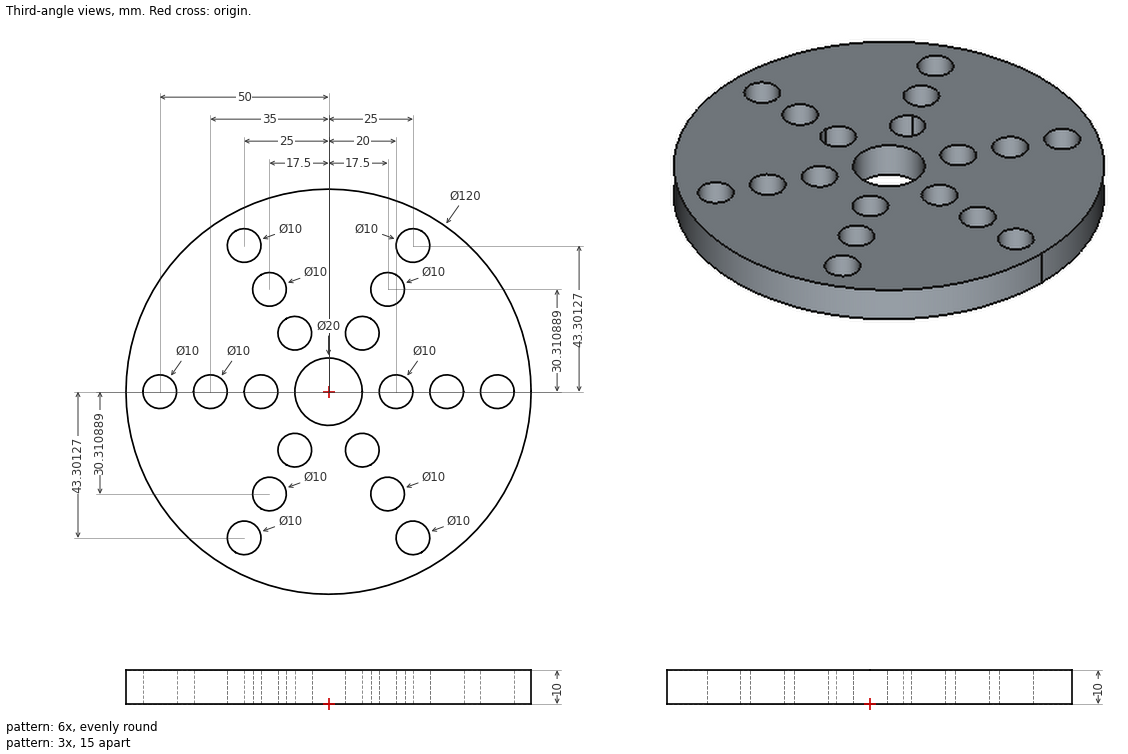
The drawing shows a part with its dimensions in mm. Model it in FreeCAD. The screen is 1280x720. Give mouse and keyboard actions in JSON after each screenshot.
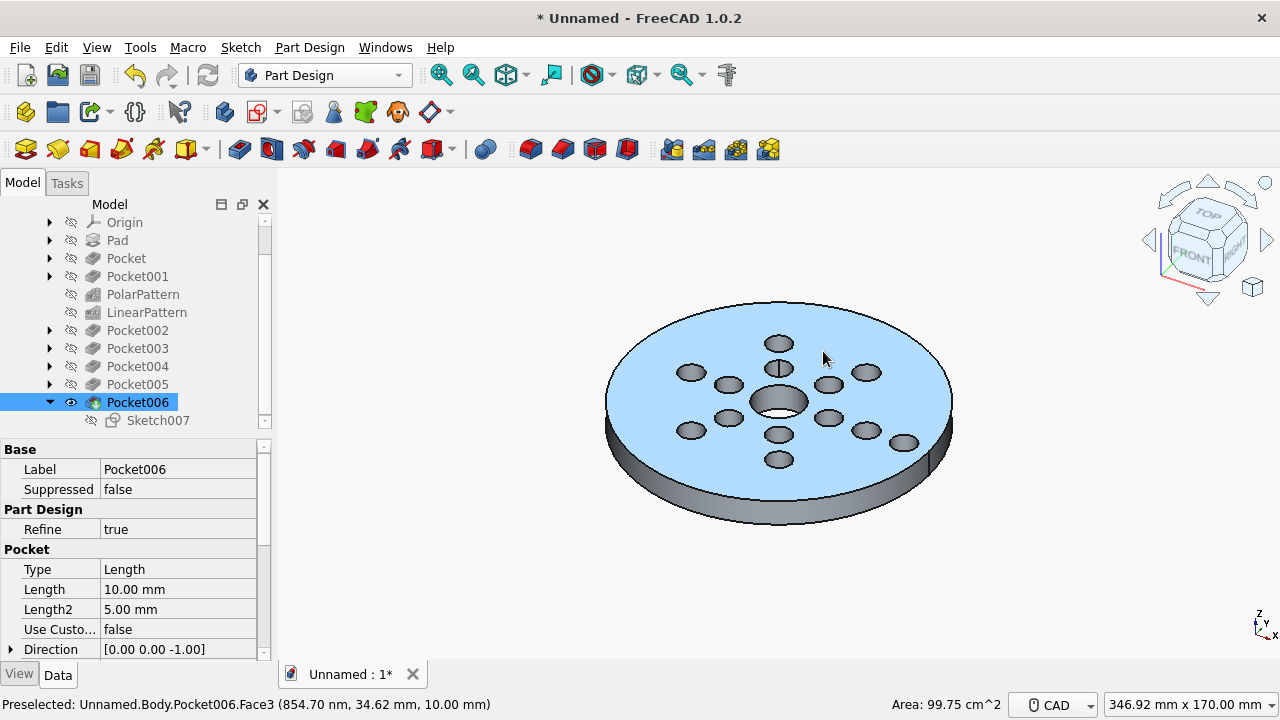
{"action": "left_click", "coordinate": [258, 112]}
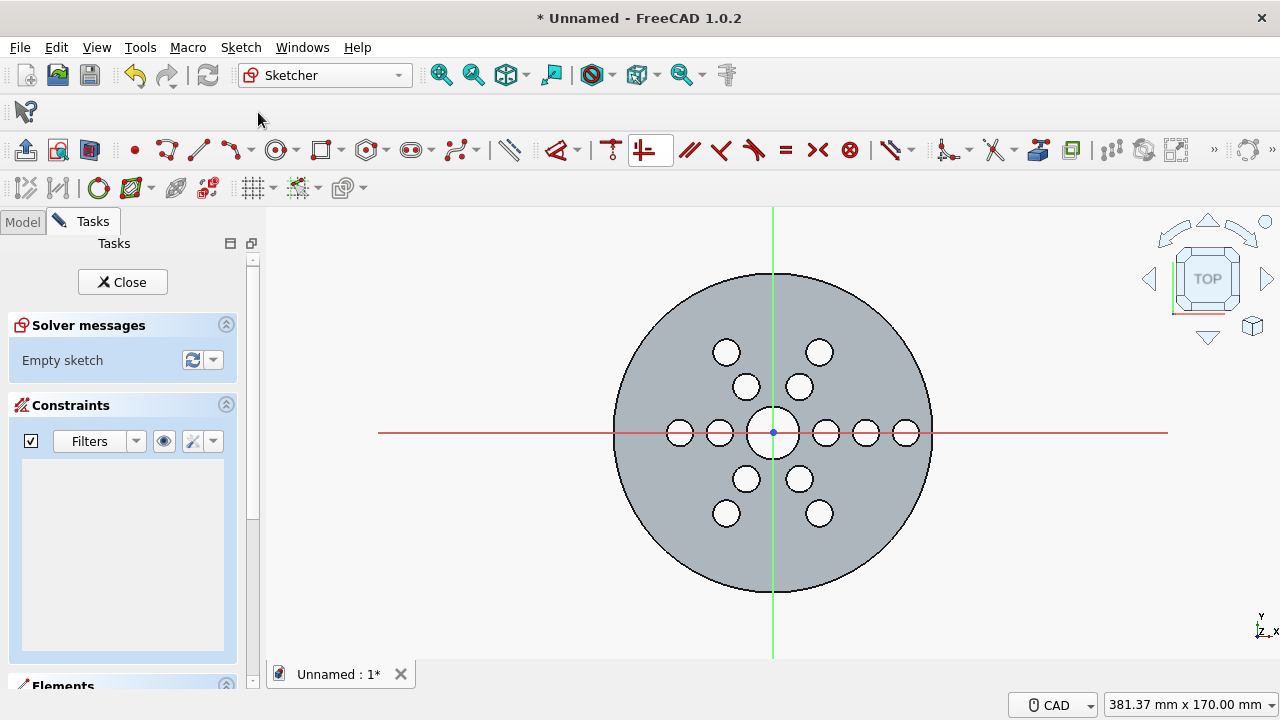
{"action": "scroll", "coordinate": [853, 306], "scroll_direction": "up", "scroll_amount": 12}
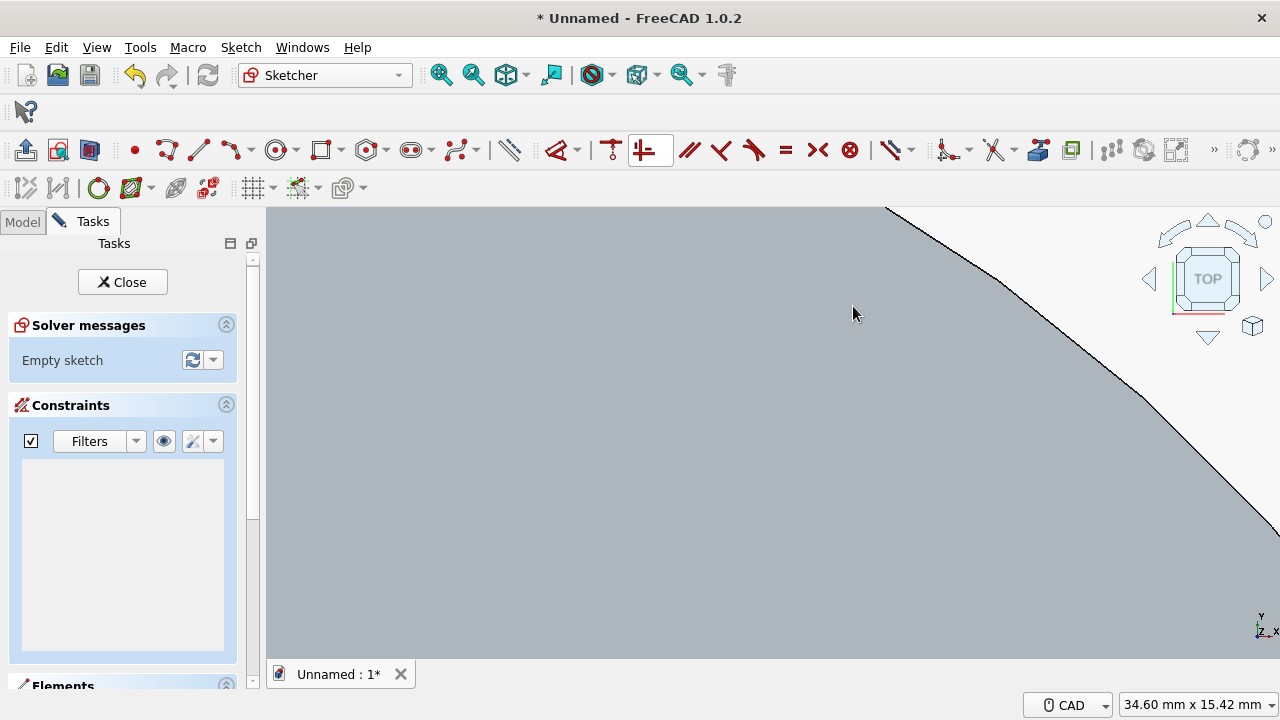
{"action": "left_click", "coordinate": [276, 150]}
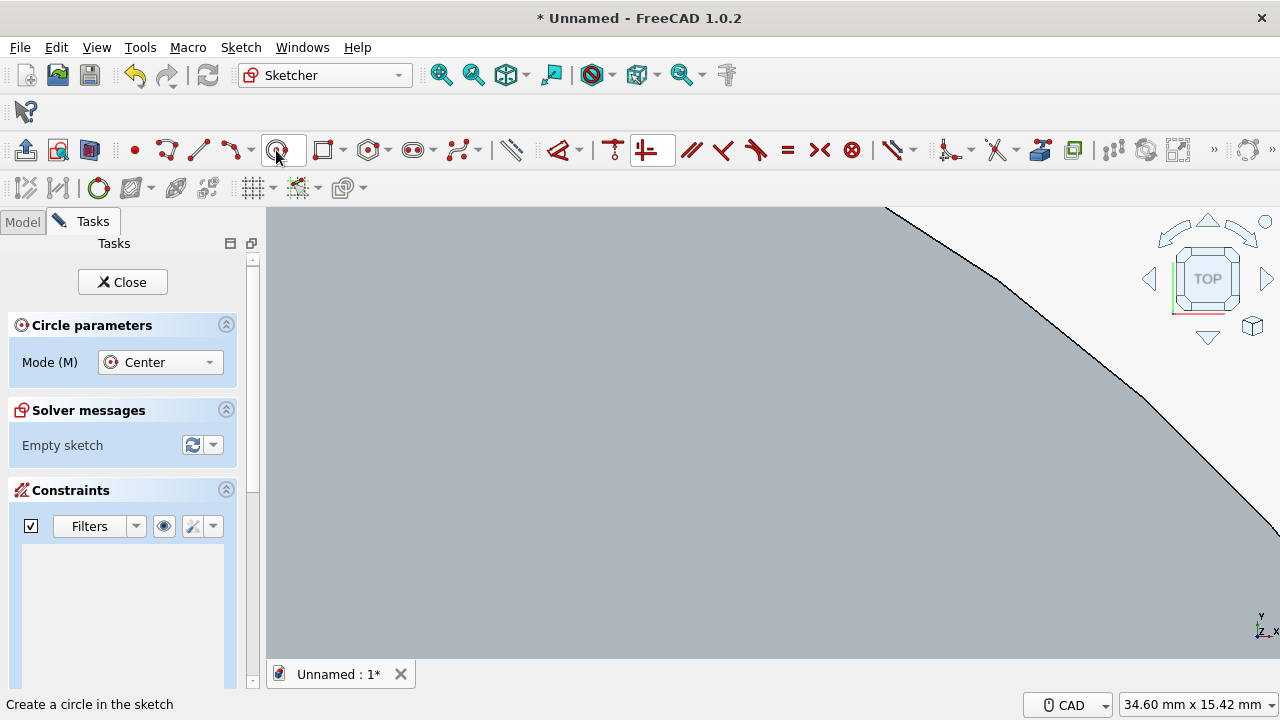
{"action": "left_click", "coordinate": [698, 435]}
{"action": "left_click", "coordinate": [802, 331]}
{"action": "key", "text": "Escape"}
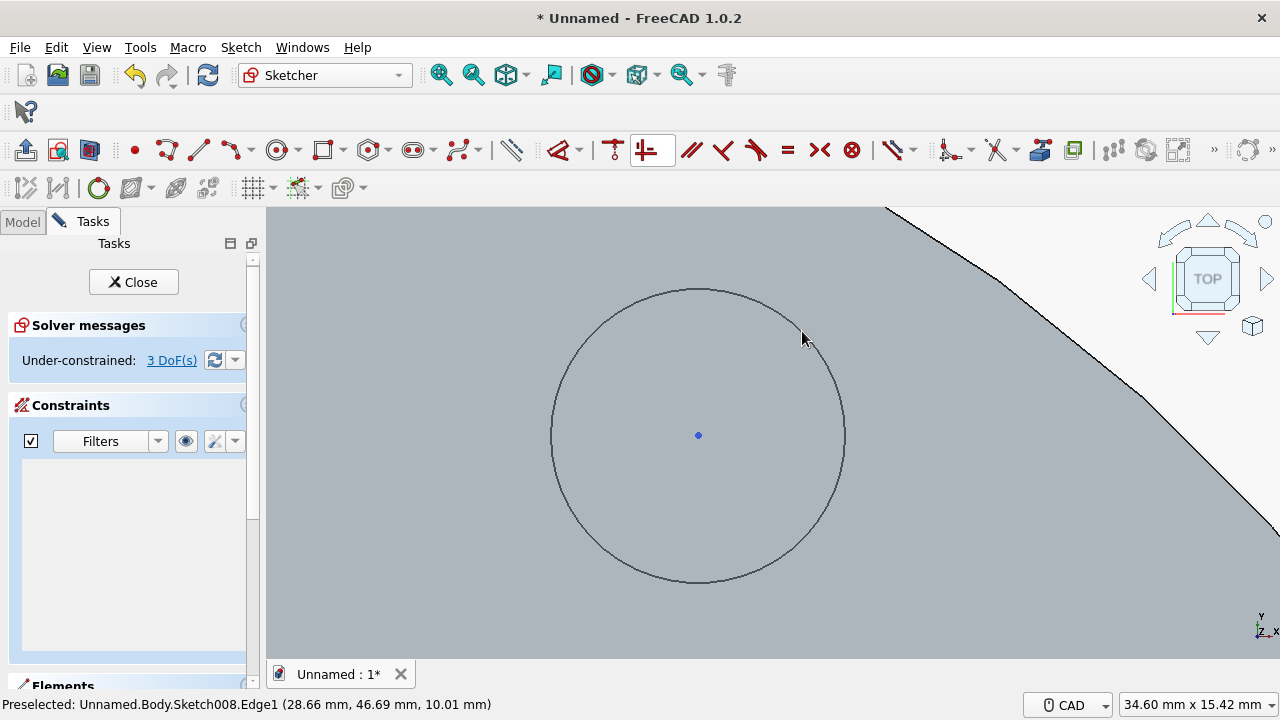
{"action": "left_click", "coordinate": [558, 150]}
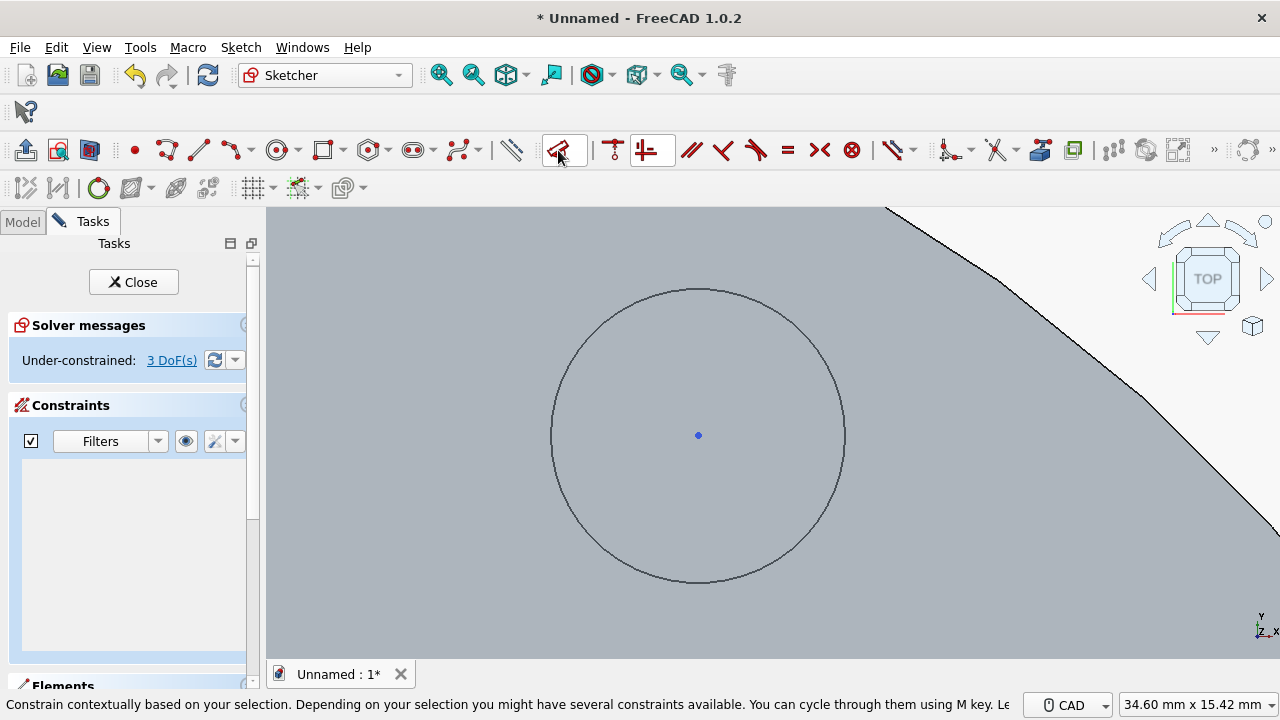
{"action": "left_click", "coordinate": [802, 332]}
{"action": "left_click", "coordinate": [825, 309]}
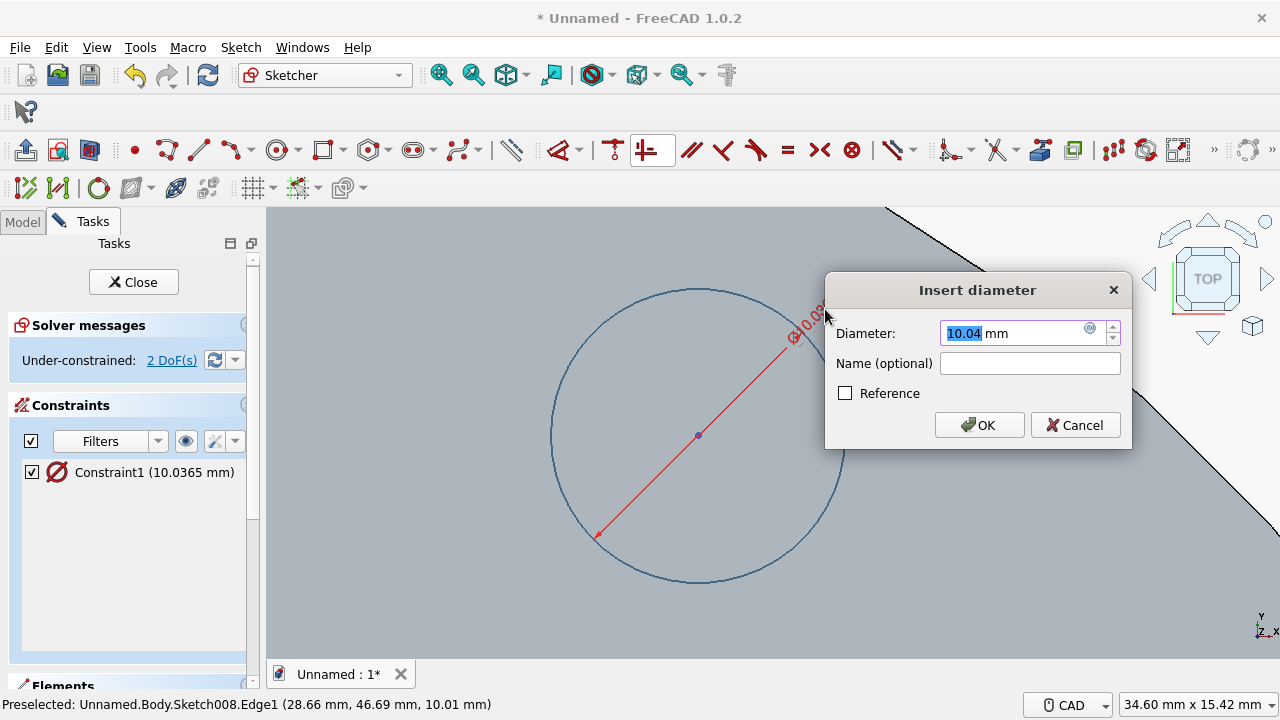
{"action": "type", "text": "10"}
{"action": "key", "text": "Return"}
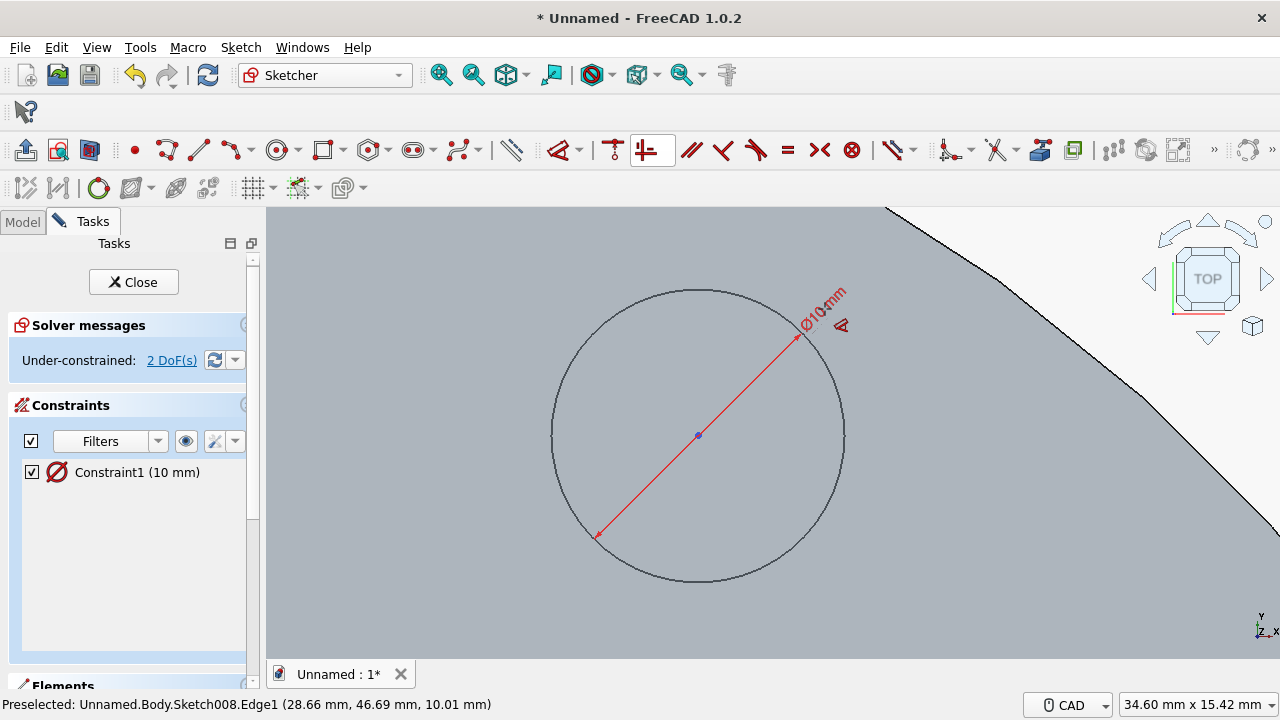
{"action": "left_click", "coordinate": [698, 436]}
{"action": "left_click", "coordinate": [496, 402]}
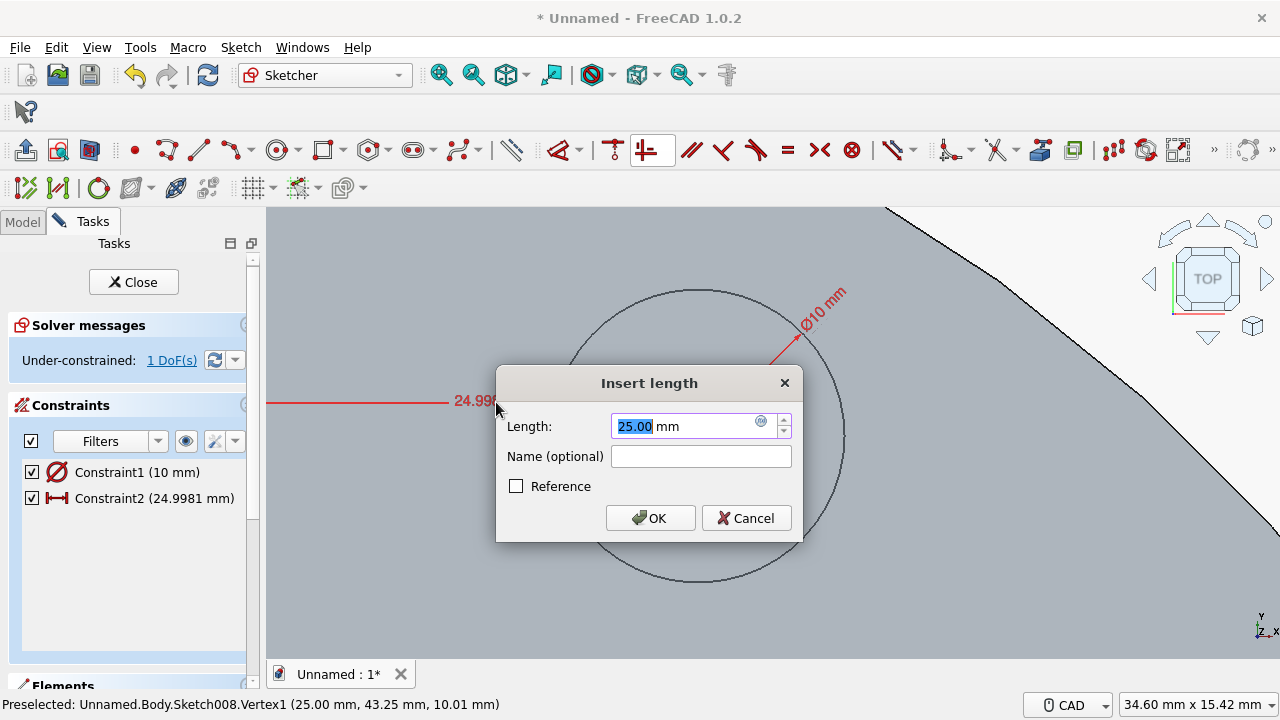
{"action": "type", "text": "25"}
{"action": "key", "text": "Return"}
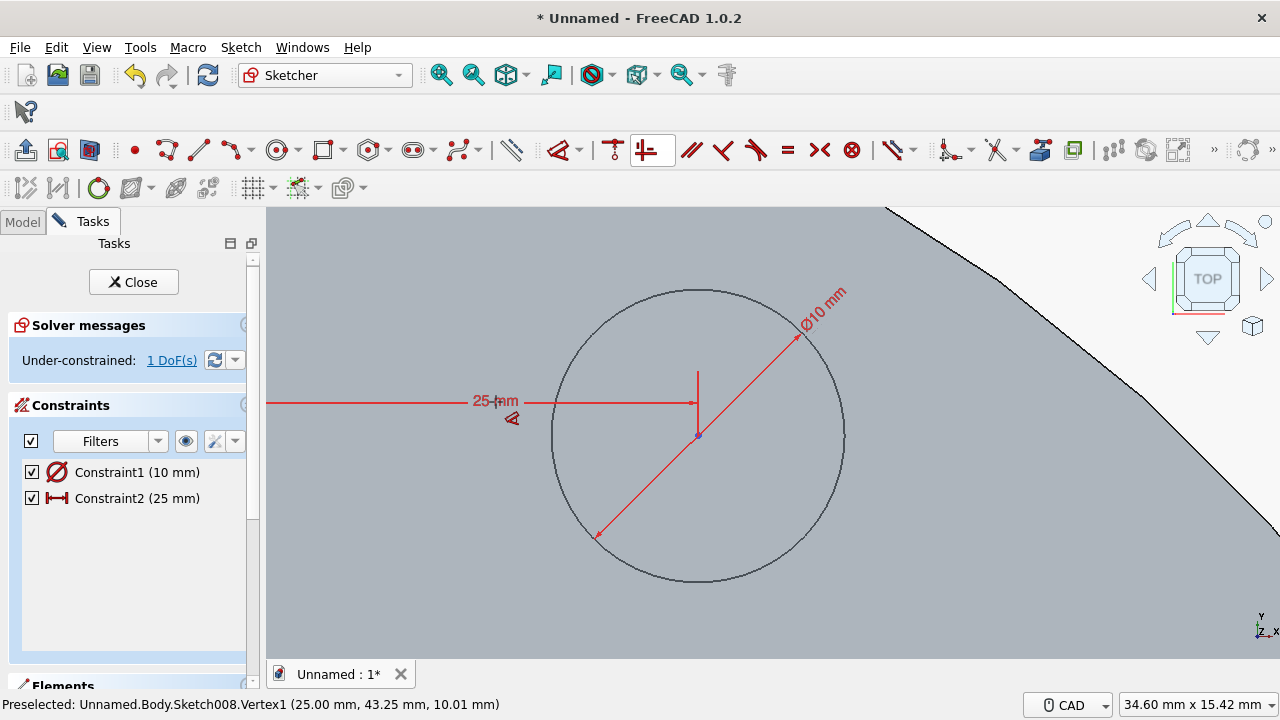
{"action": "left_click", "coordinate": [698, 436]}
{"action": "left_click", "coordinate": [732, 534]}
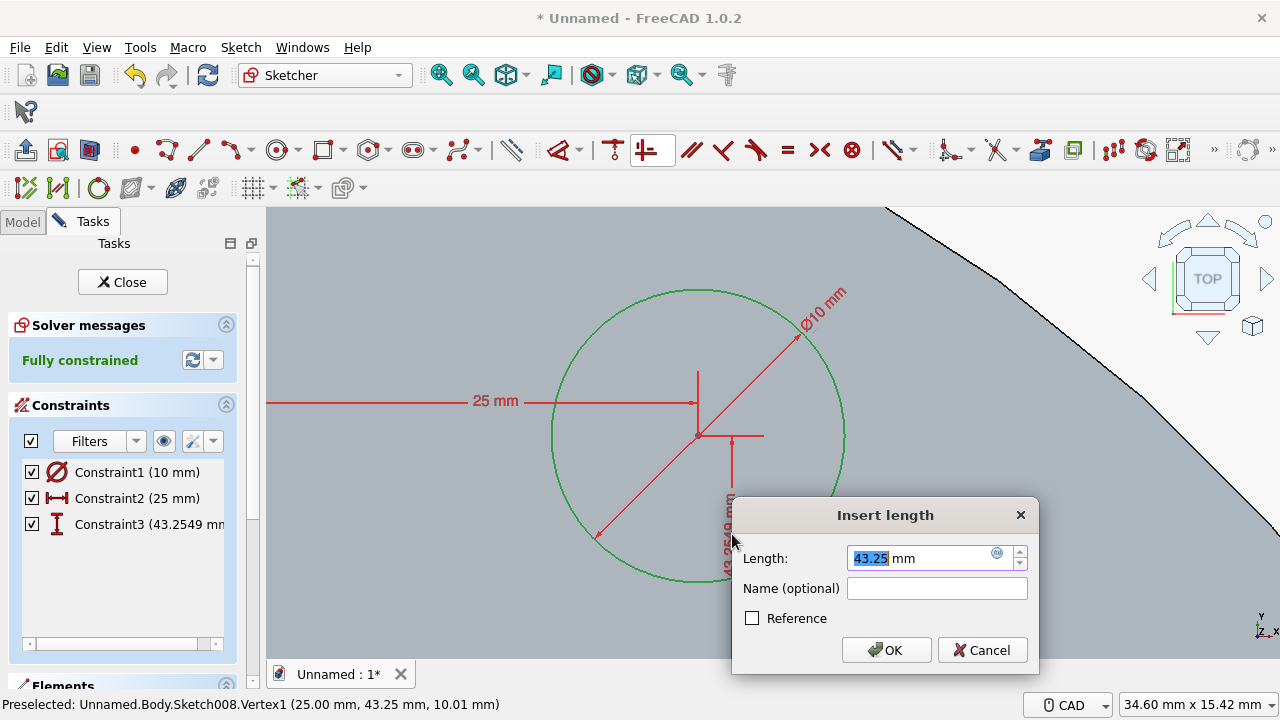
{"action": "type", "text": "43.30127"}
{"action": "key", "text": "Return"}
{"action": "key", "text": "Escape"}